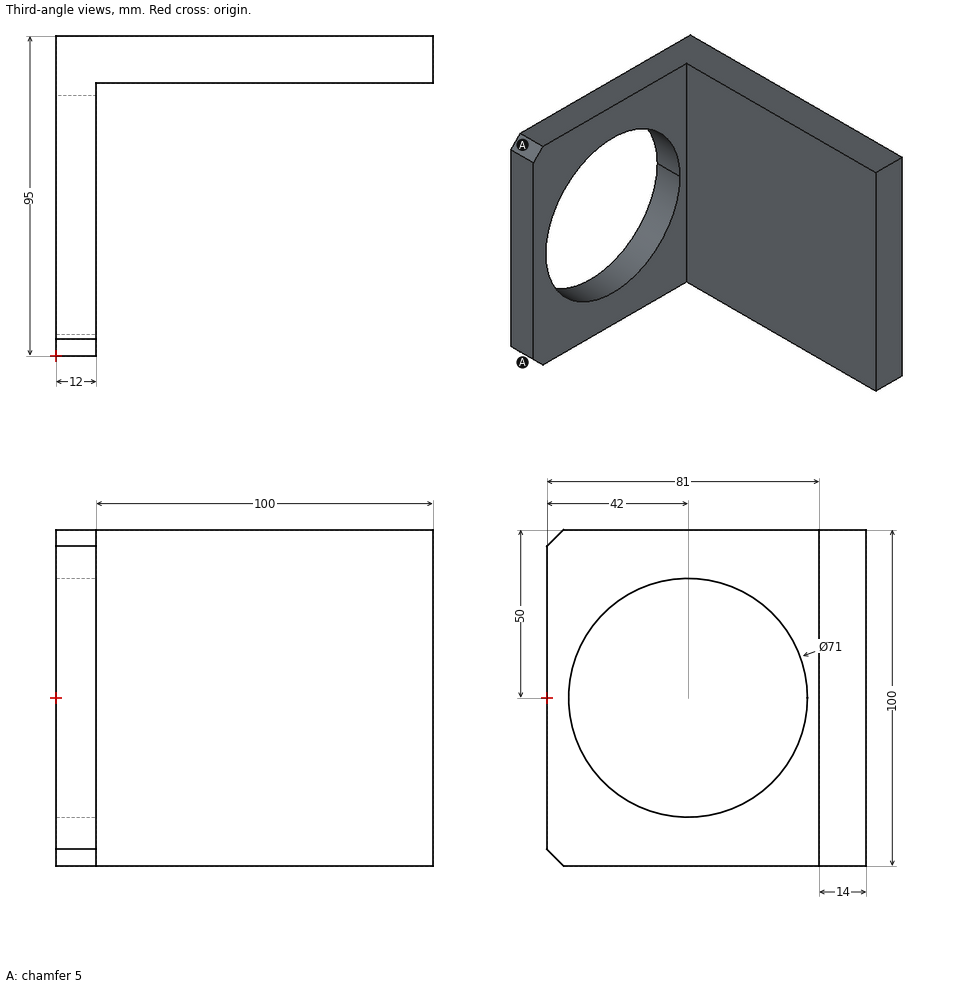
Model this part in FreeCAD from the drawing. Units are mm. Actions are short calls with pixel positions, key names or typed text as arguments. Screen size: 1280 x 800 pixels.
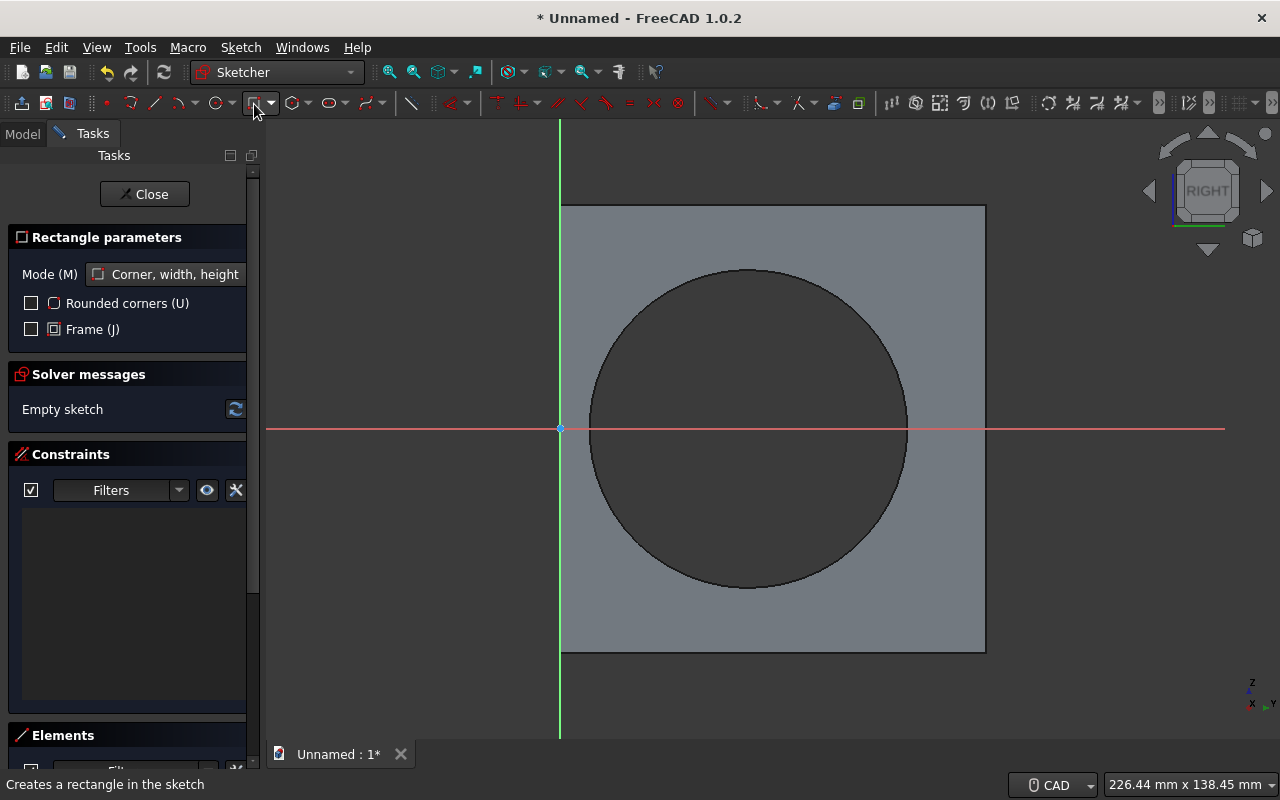
click(923, 205)
move(986, 653)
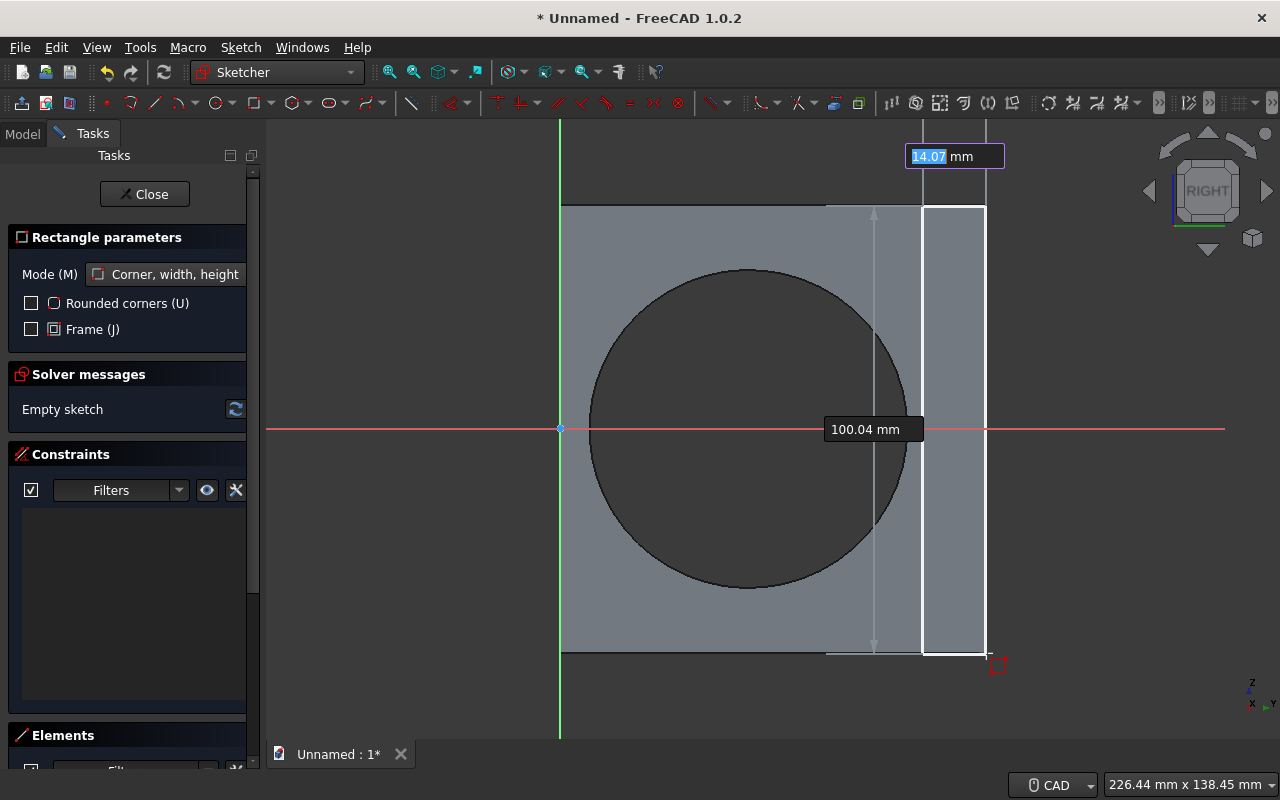
text(14)
key(Tab)
text(100)
key(Return)
key(Escape)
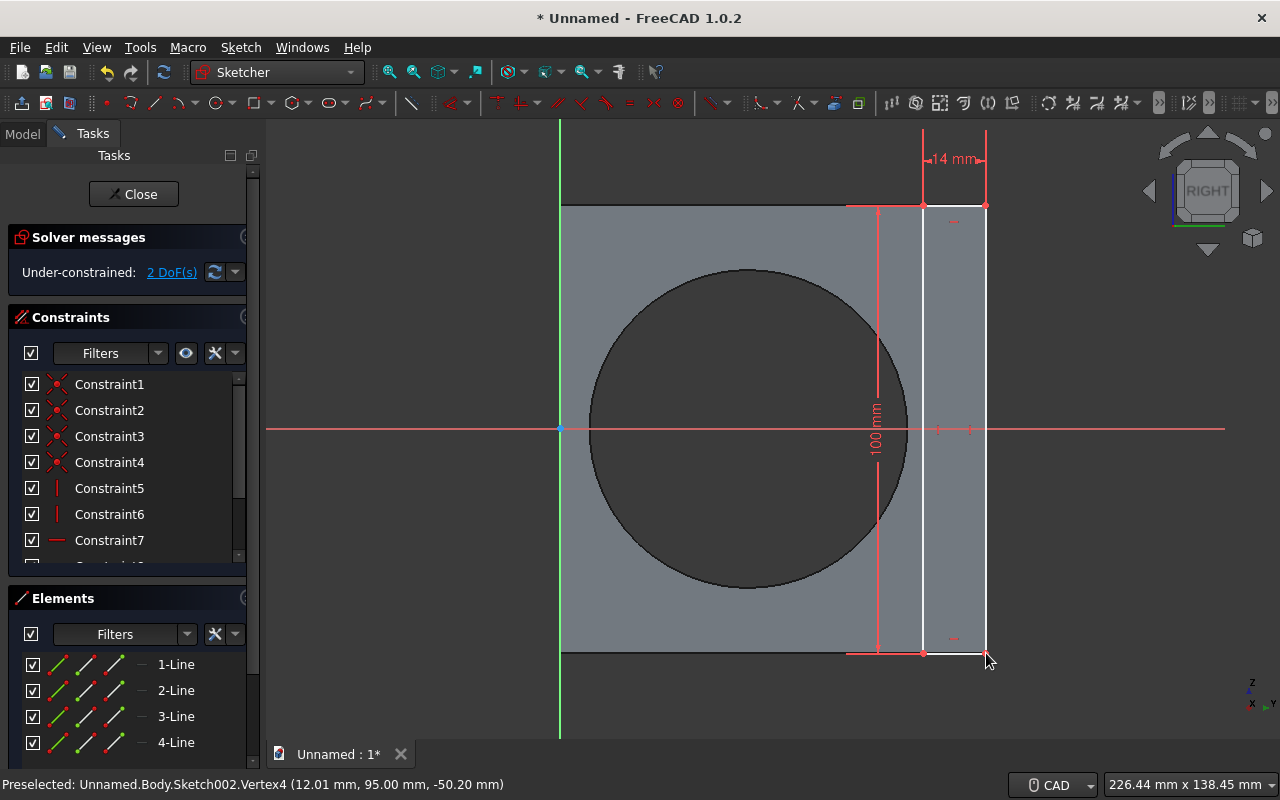
click(450, 104)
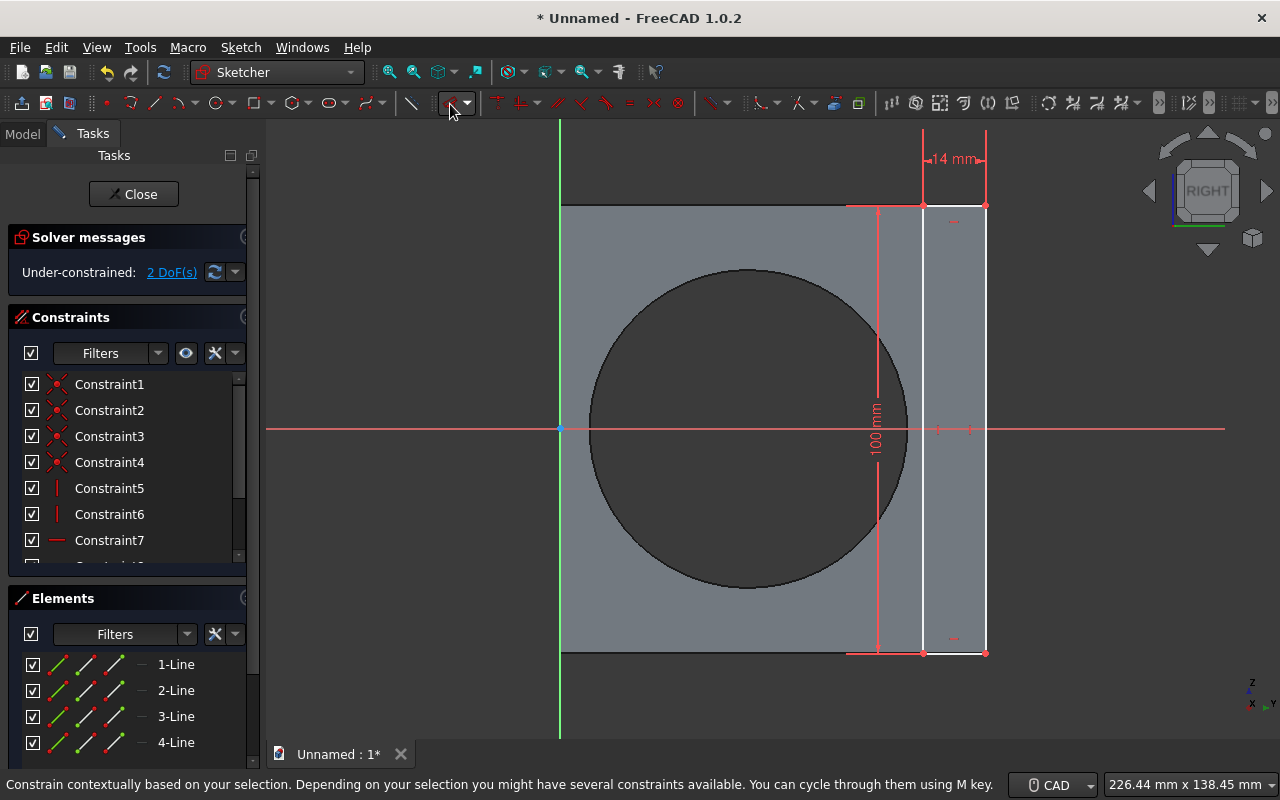
click(923, 206)
click(742, 172)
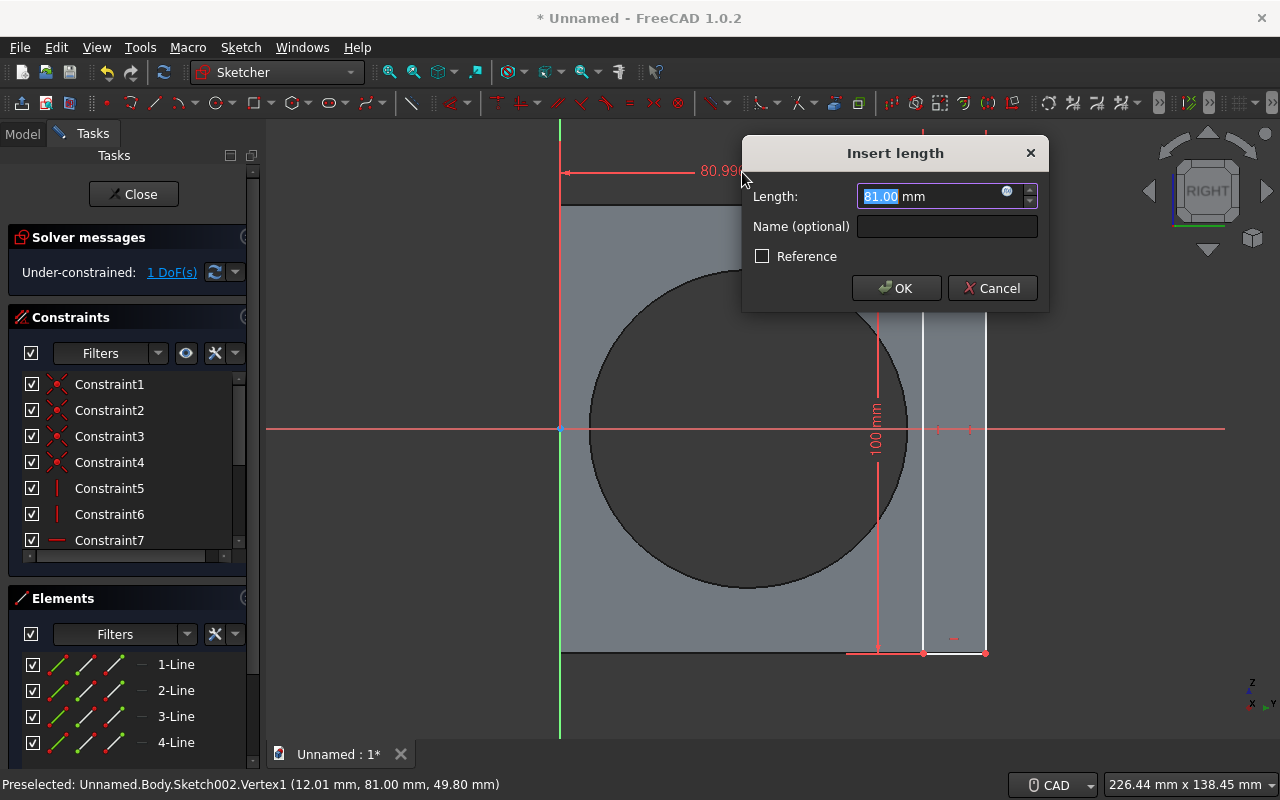
text(81)
key(Return)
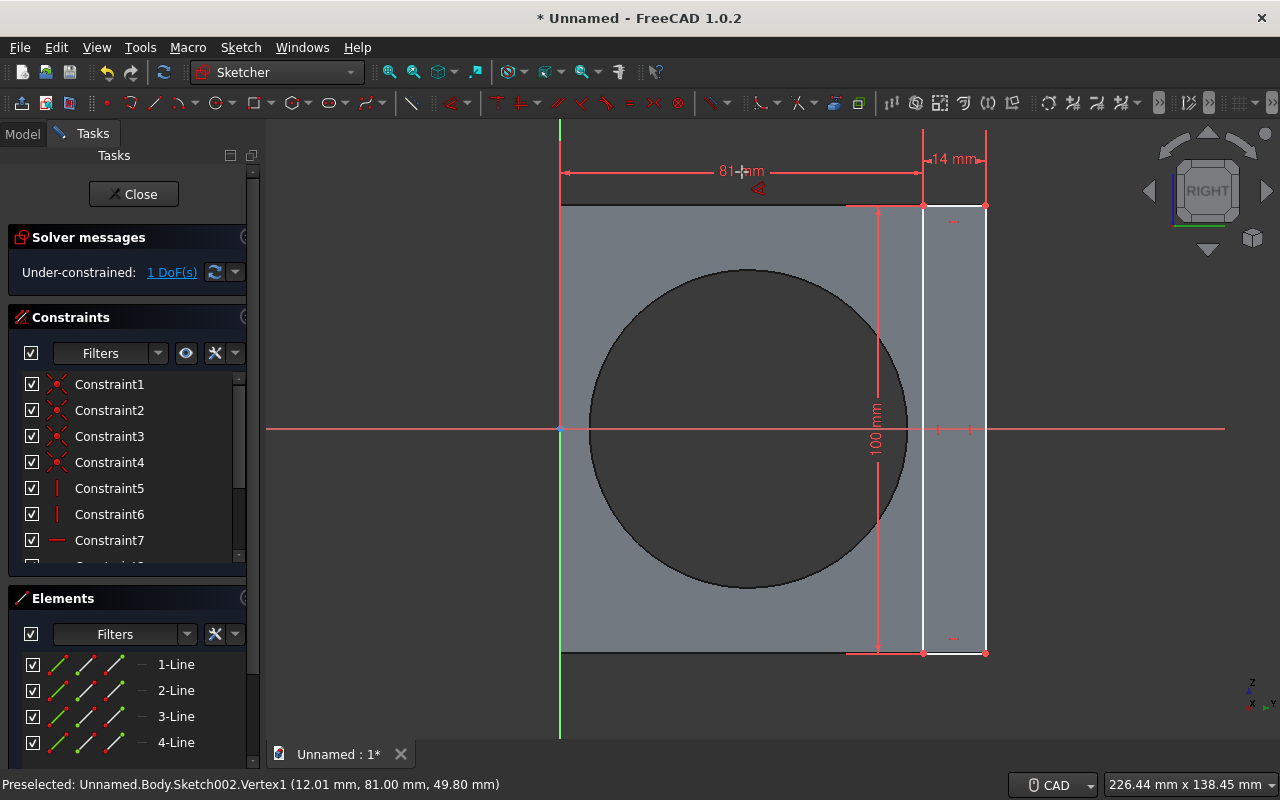
click(923, 206)
click(526, 317)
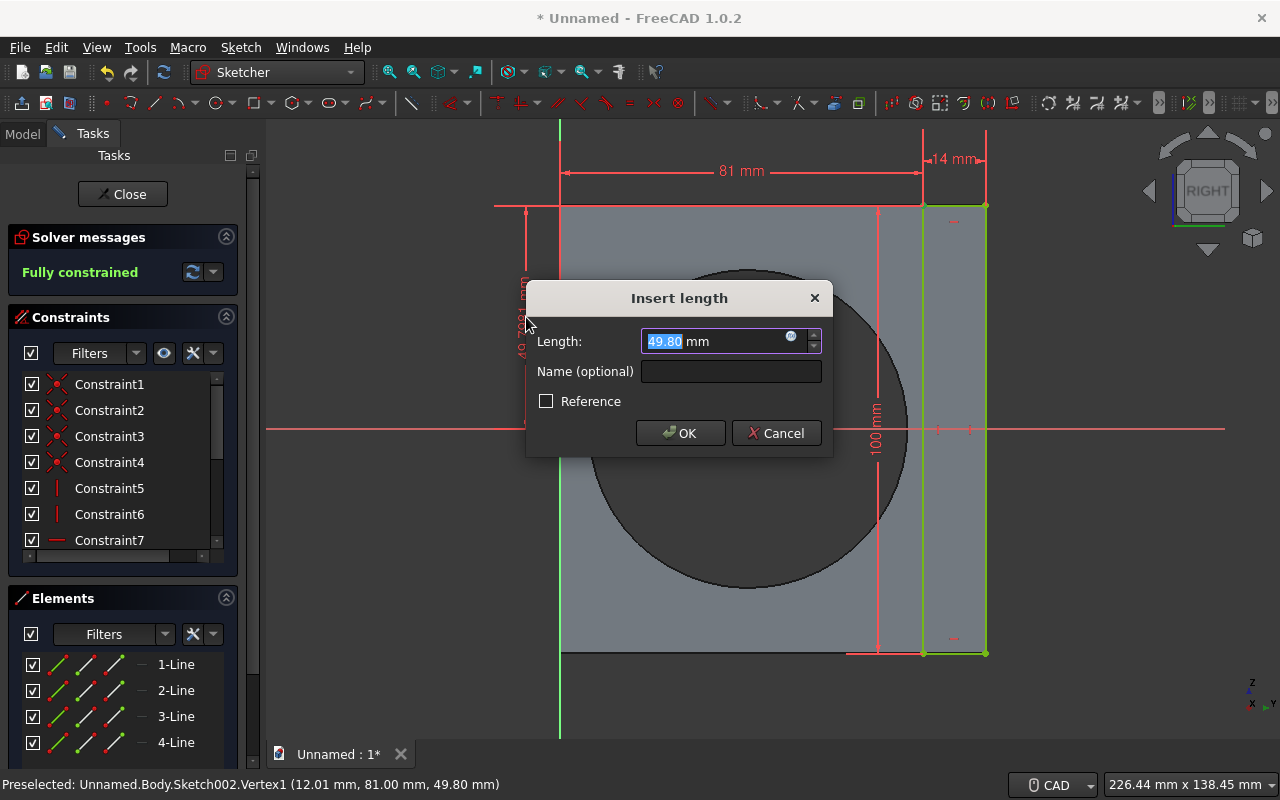
text(50)
key(Return)
key(Escape)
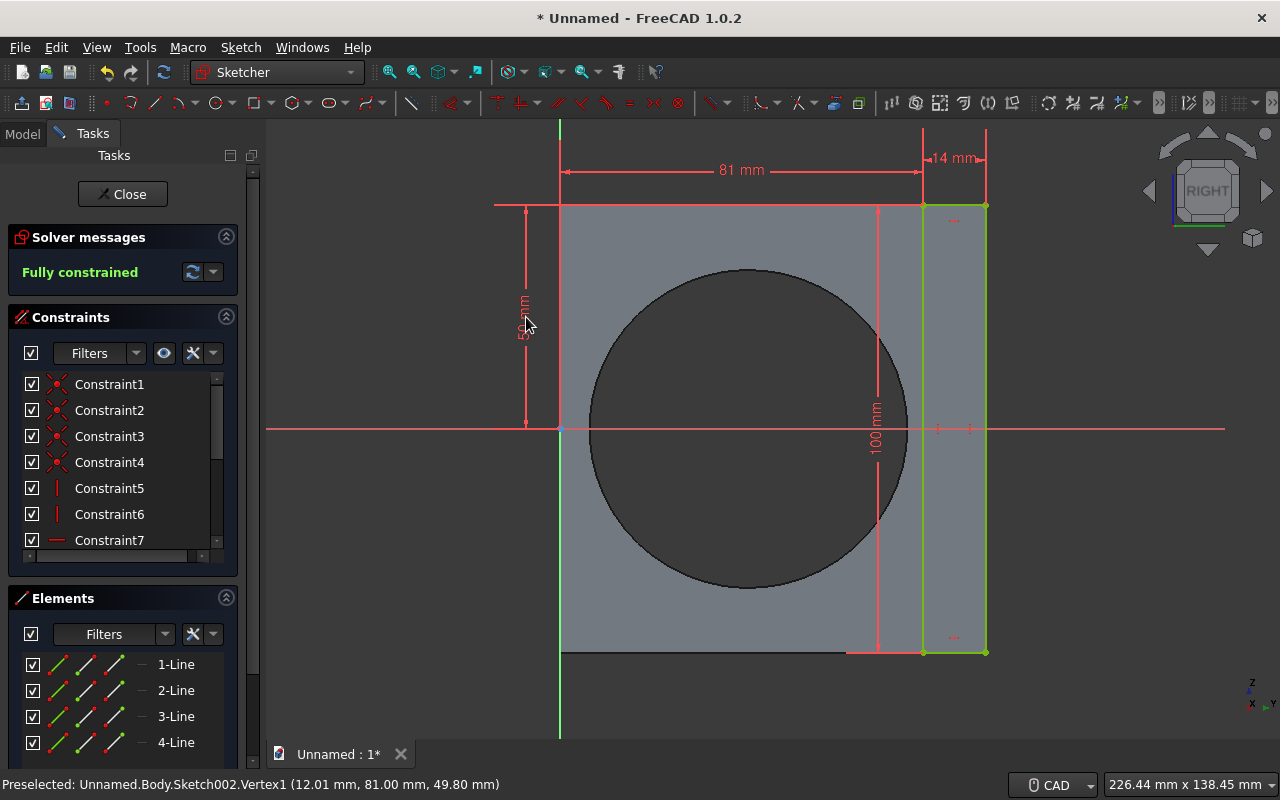
click(123, 194)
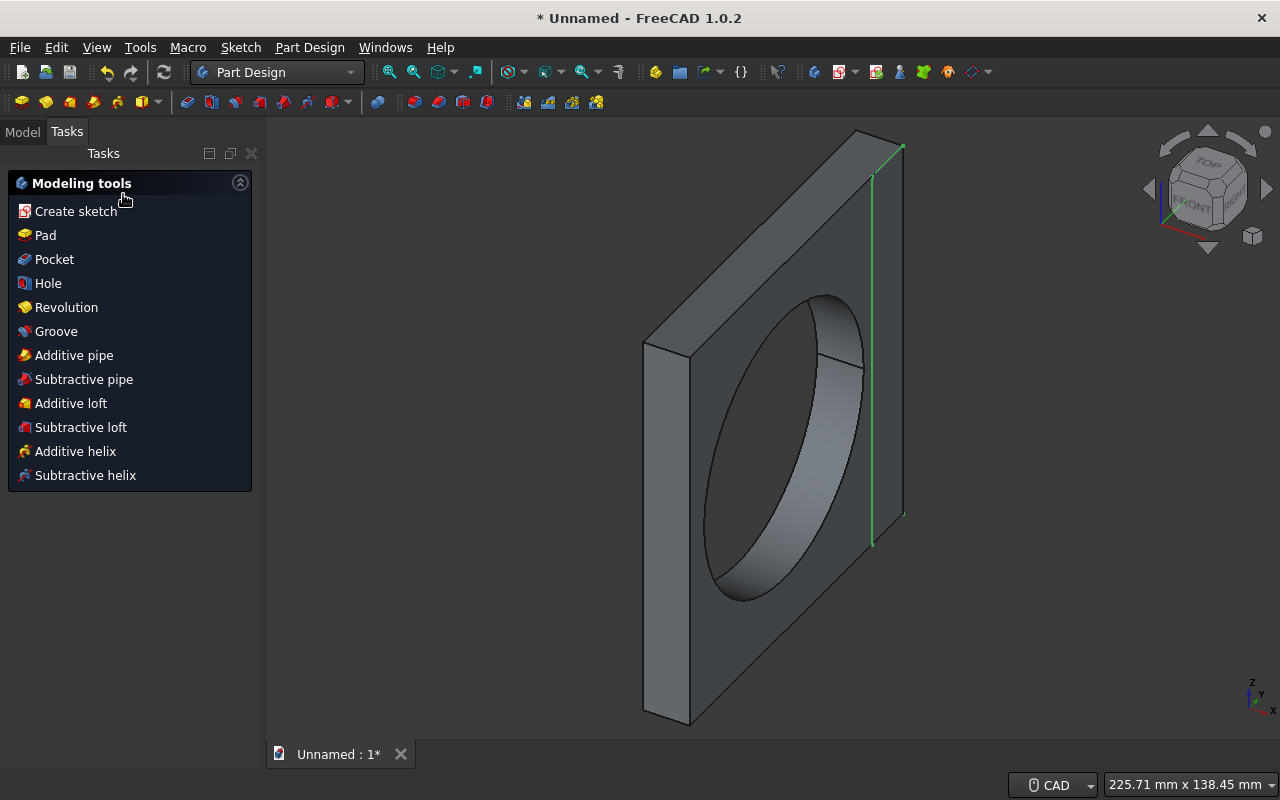
click(22, 102)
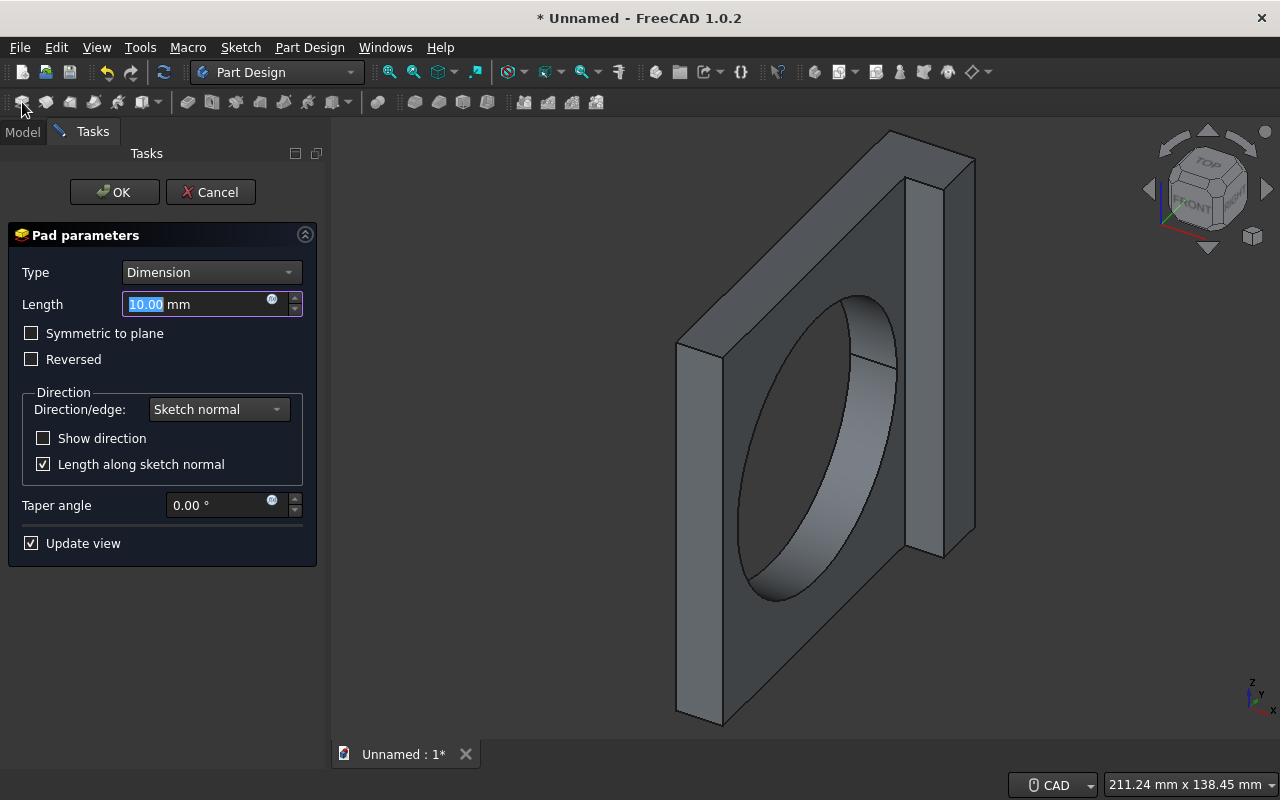
text(100)
key(Tab)